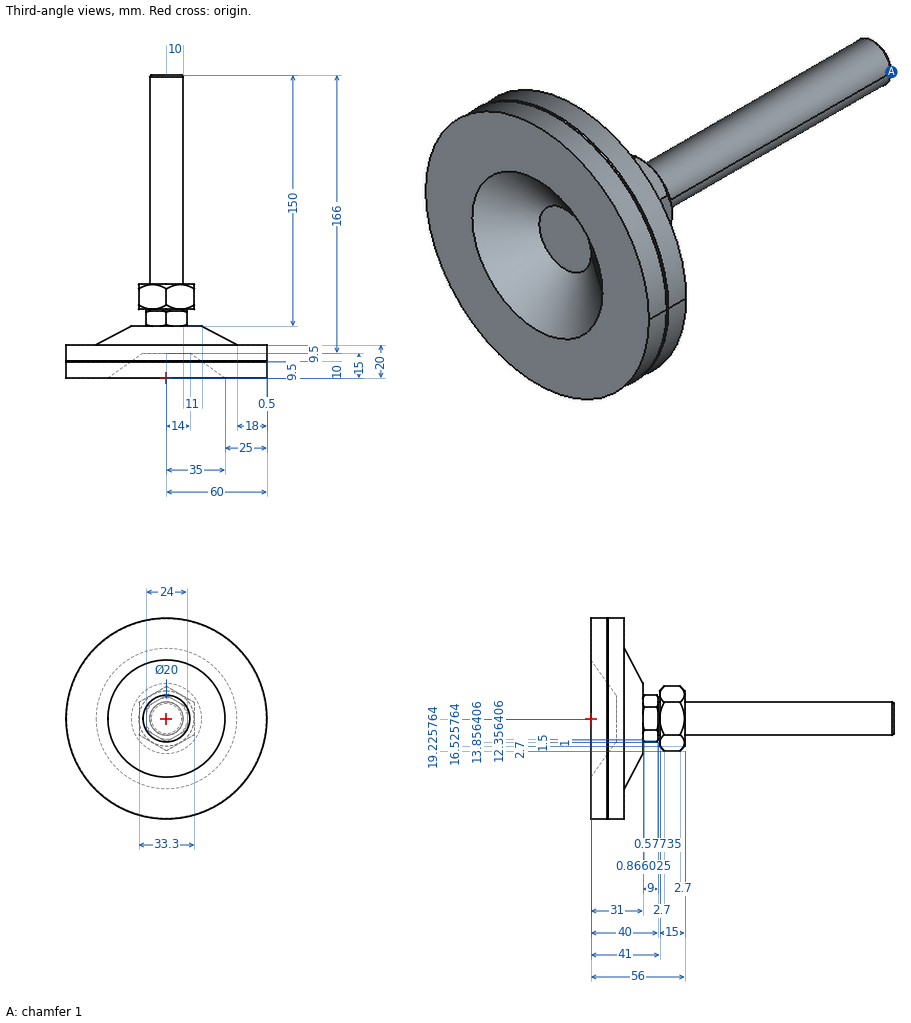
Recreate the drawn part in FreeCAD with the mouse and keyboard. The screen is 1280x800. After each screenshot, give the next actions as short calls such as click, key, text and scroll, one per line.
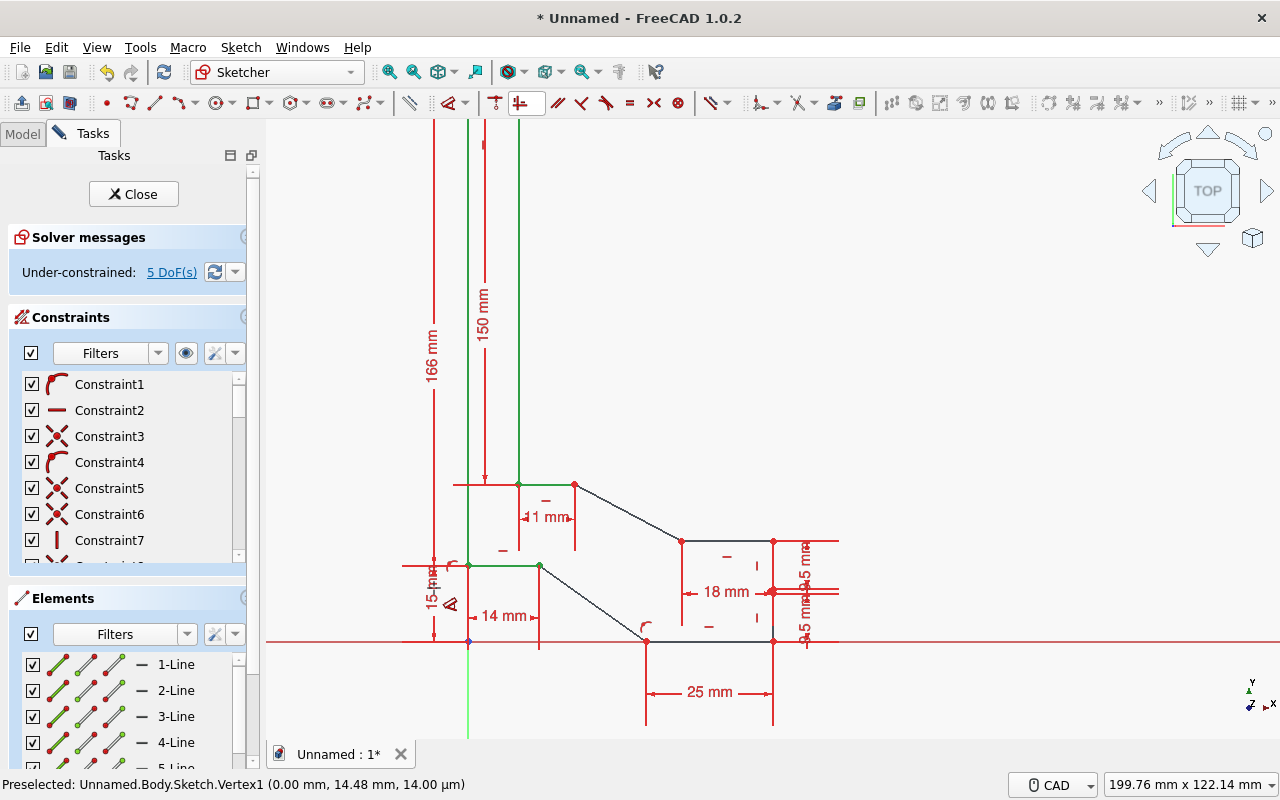
click(646, 642)
click(557, 676)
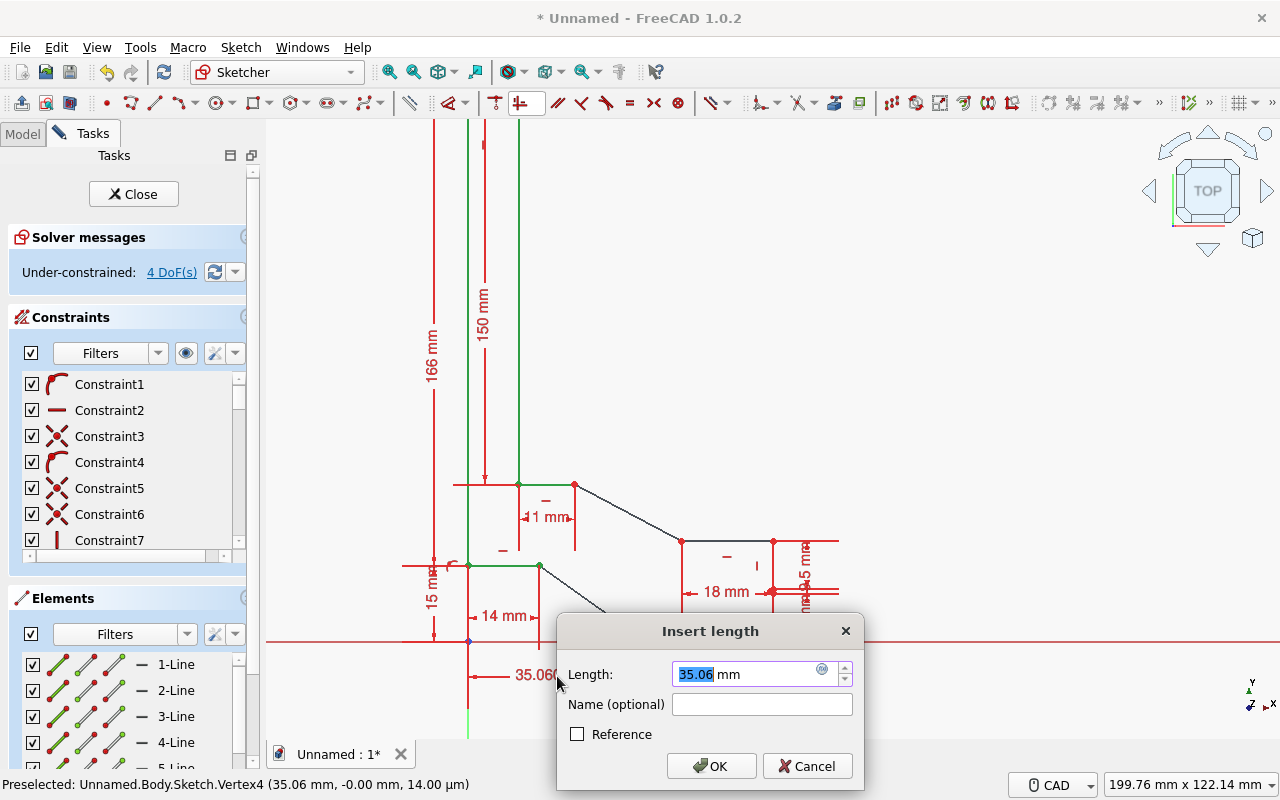
text(35)
key(Return)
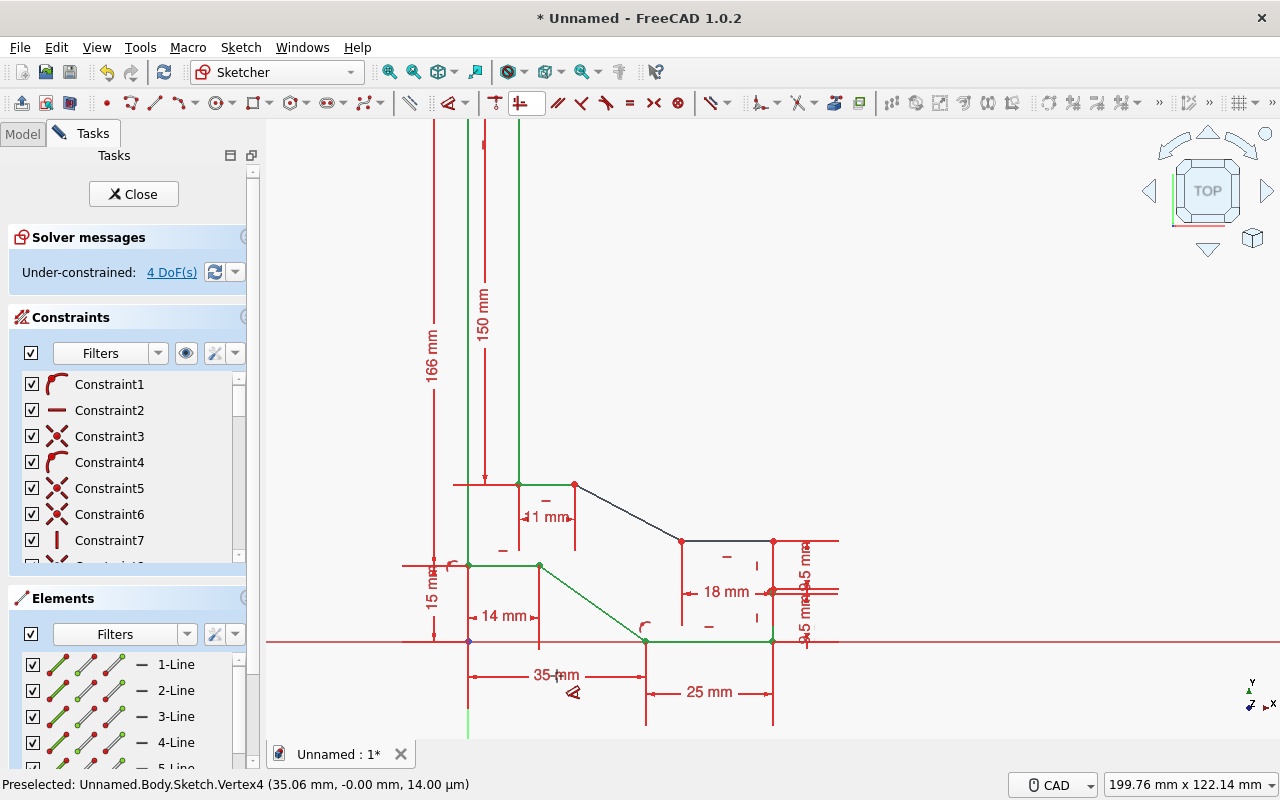
scroll(770, 591, up, 7)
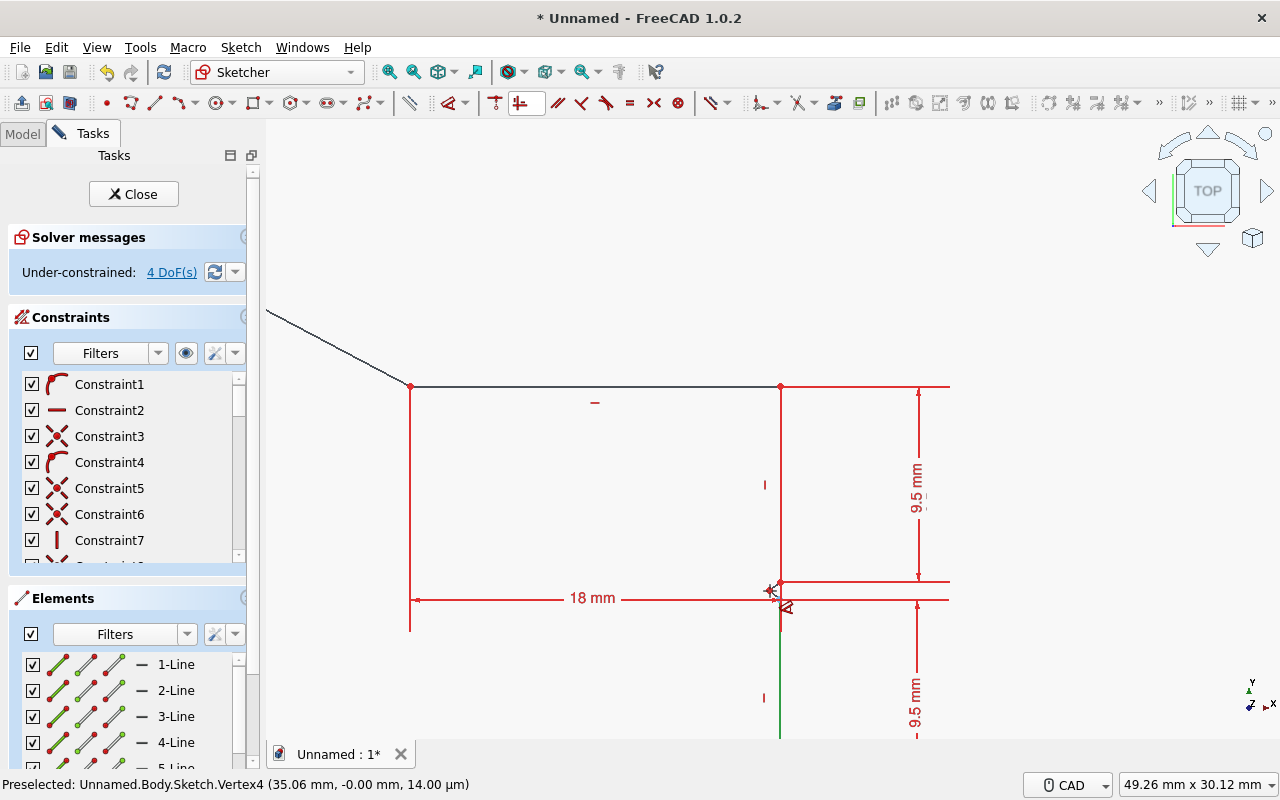
click(770, 590)
click(804, 651)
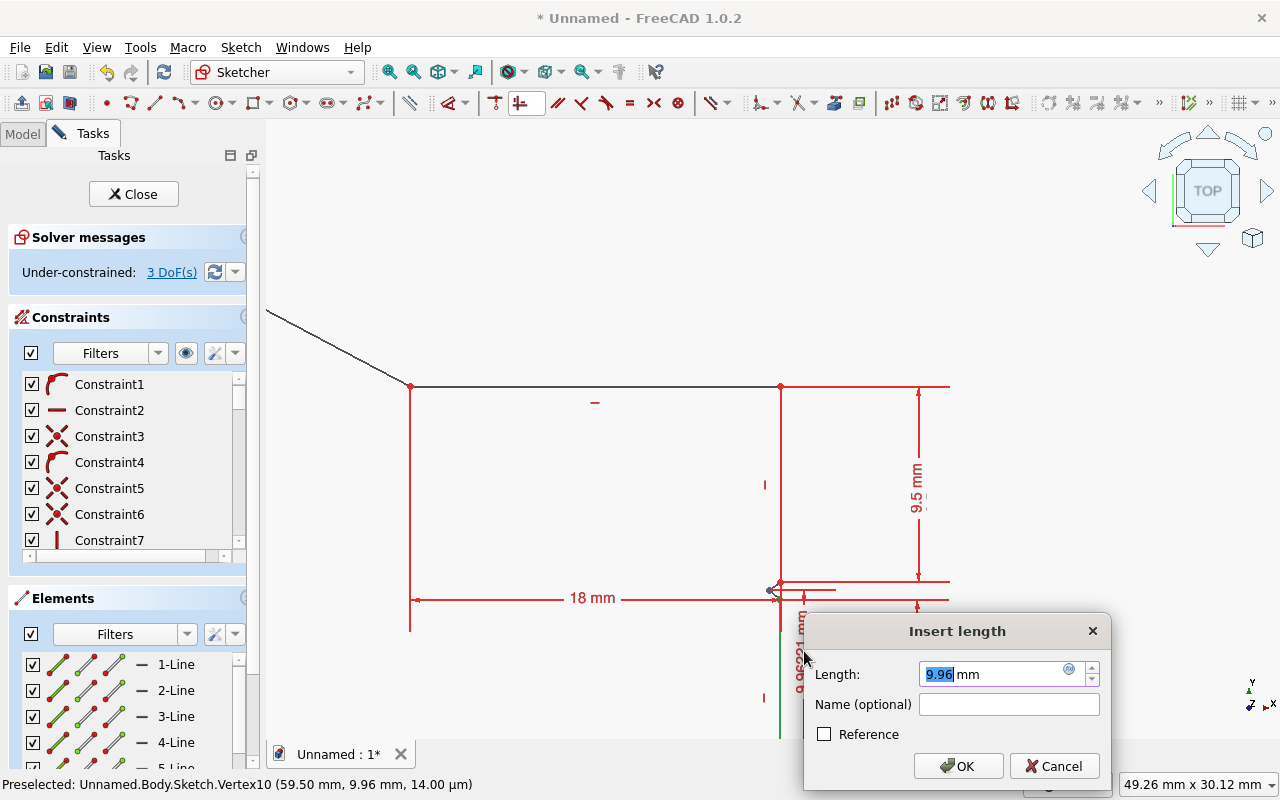
text(10)
key(Return)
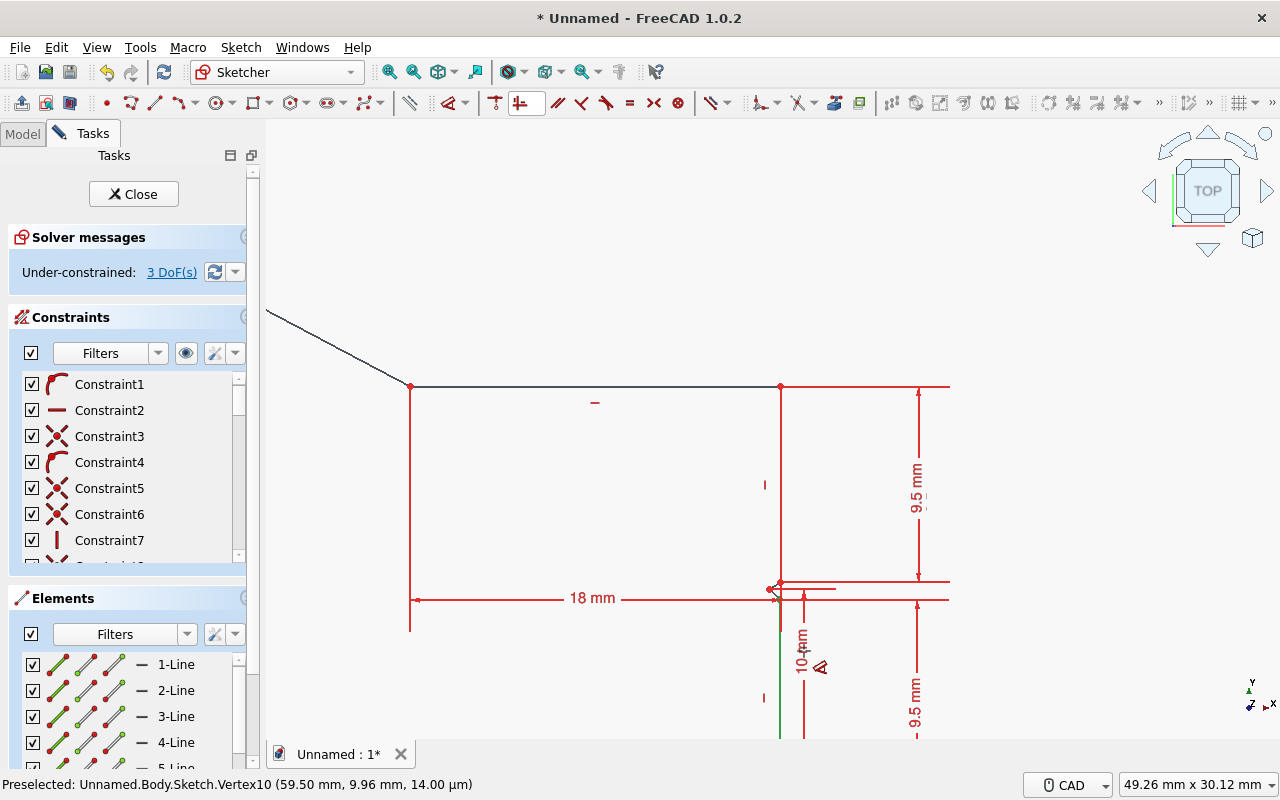
click(781, 582)
click(537, 548)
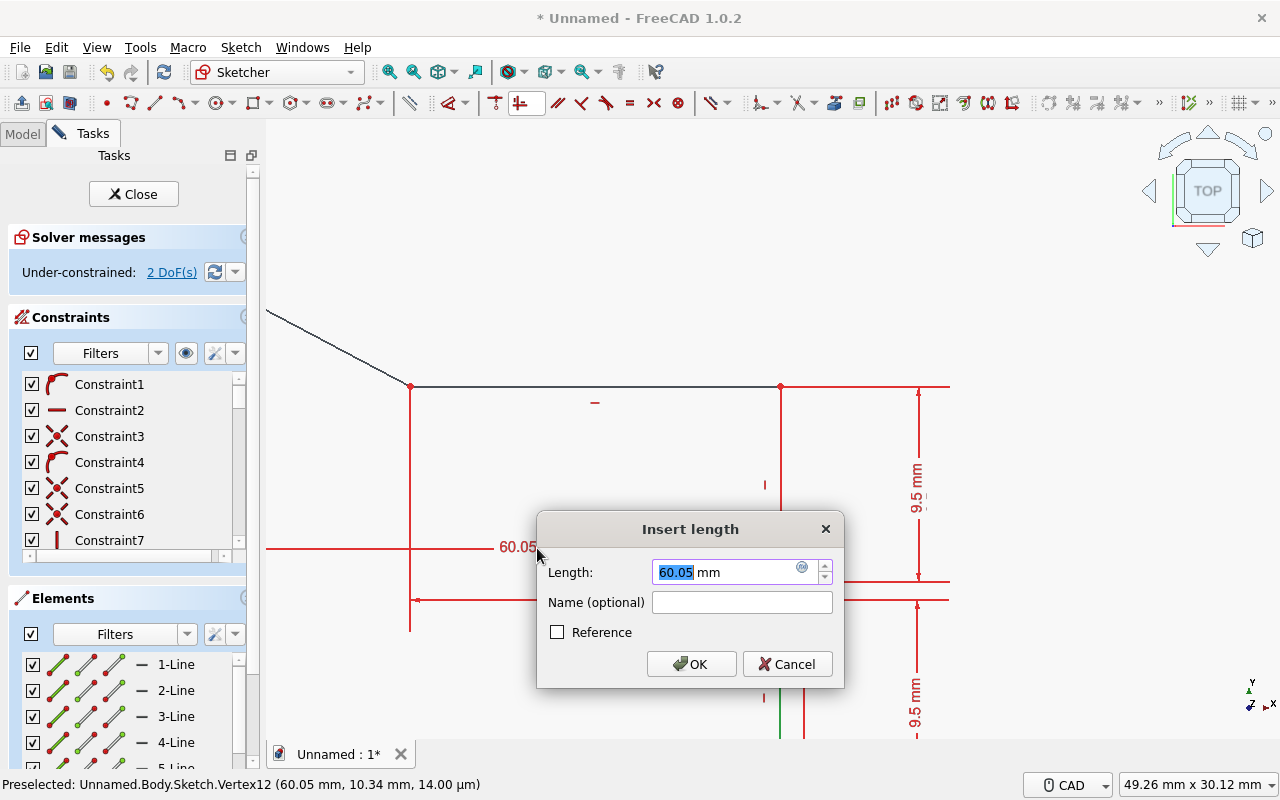
text(60)
key(Return)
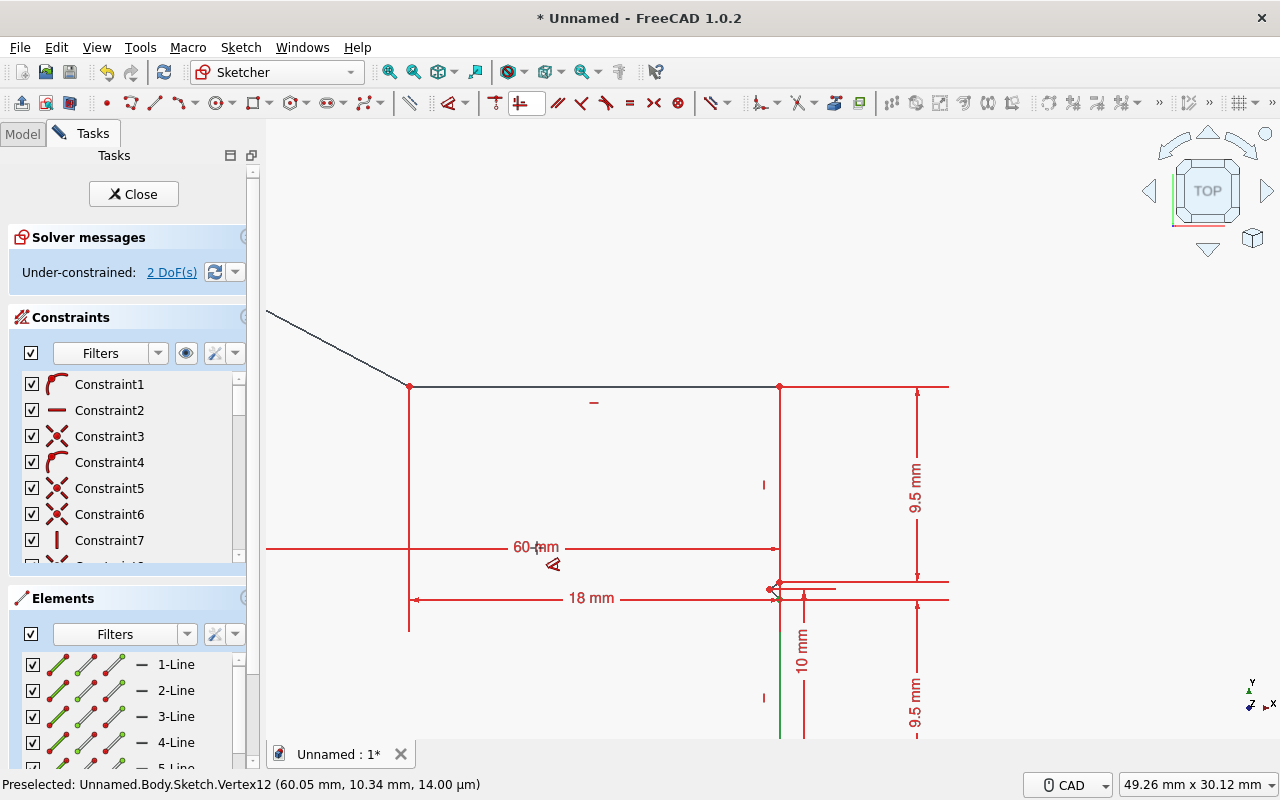
scroll(772, 616, down, 11)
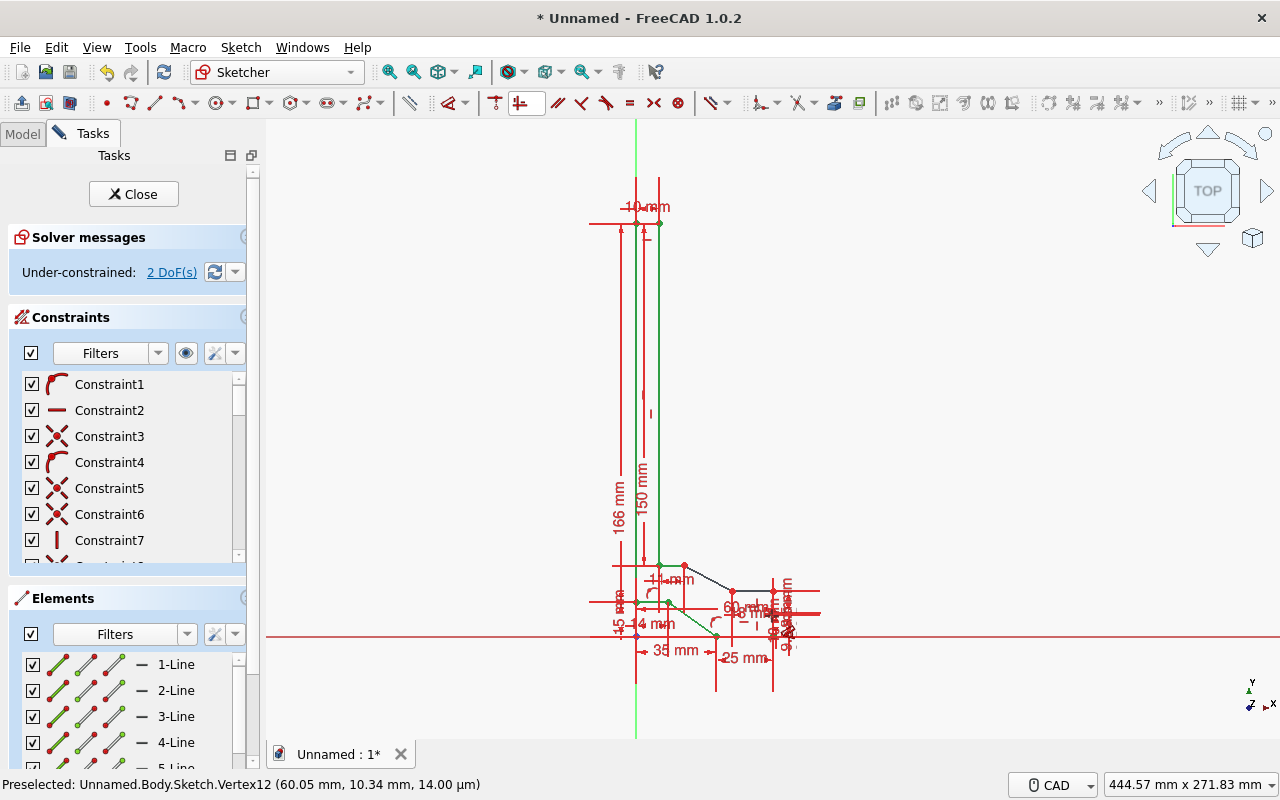
click(773, 591)
click(879, 614)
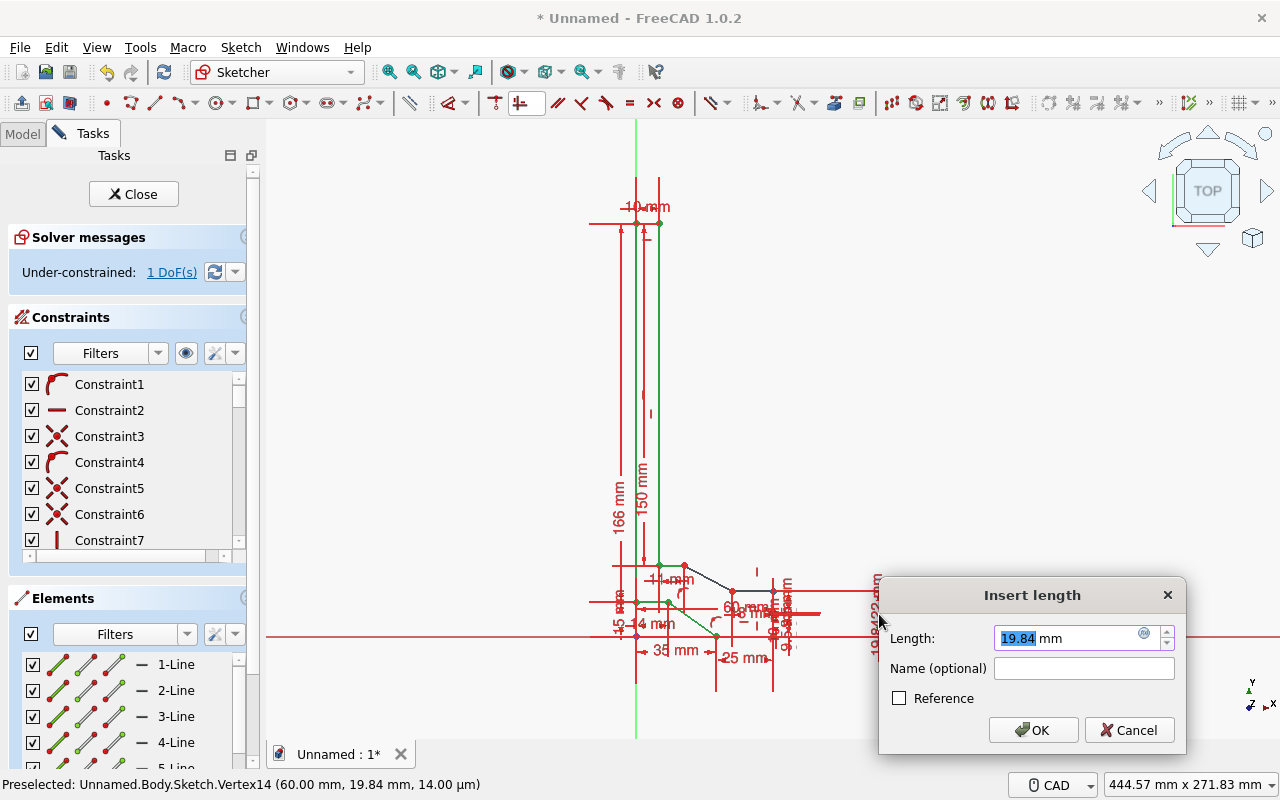
text(20)
key(Return)